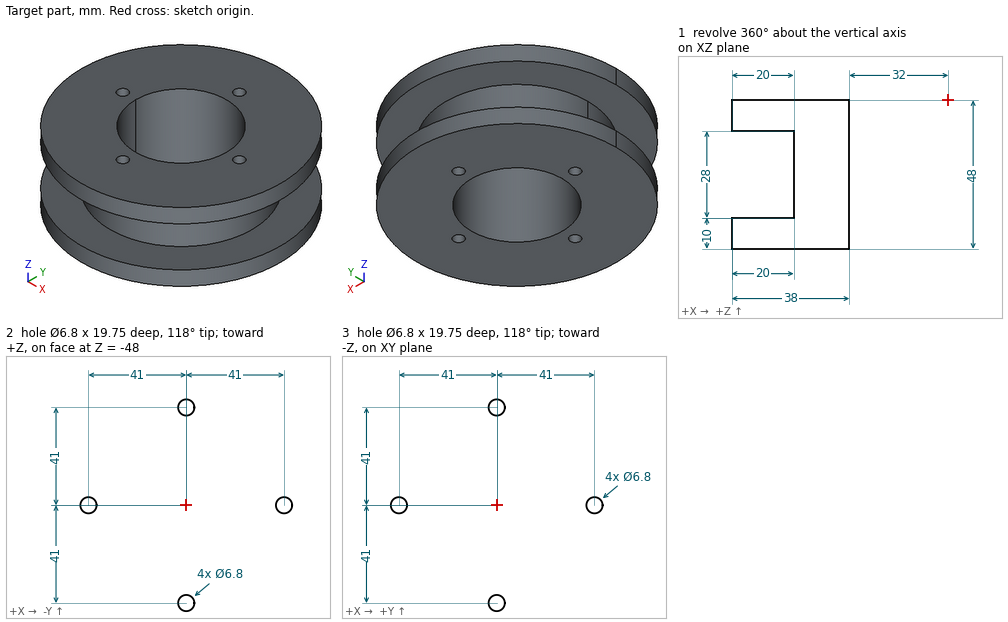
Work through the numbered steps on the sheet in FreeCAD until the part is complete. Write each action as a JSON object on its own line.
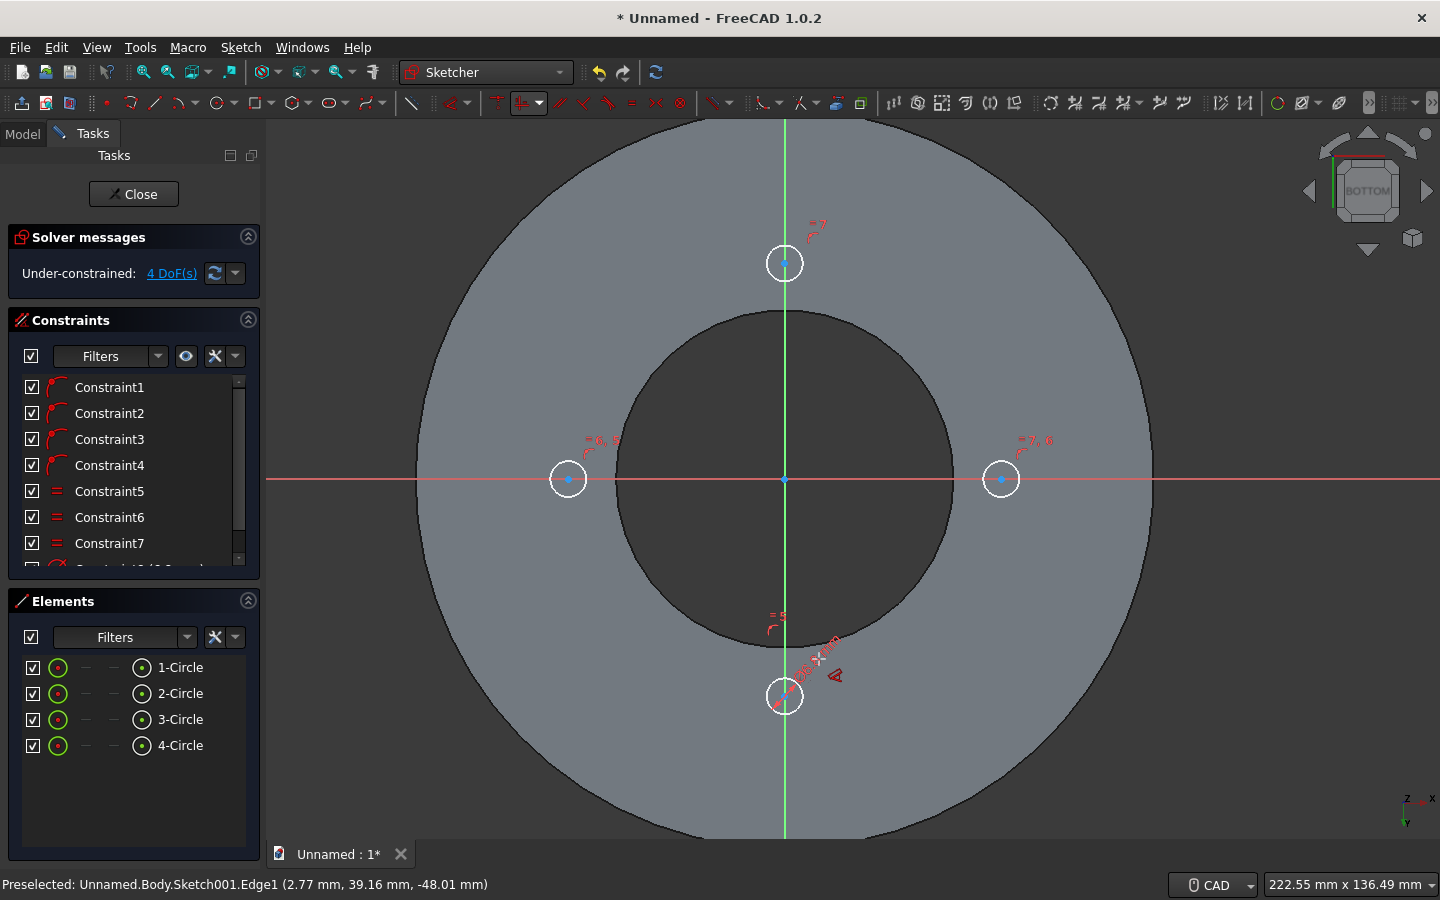
{"action": "left_click", "coordinate": [785, 696]}
{"action": "left_click", "coordinate": [819, 588]}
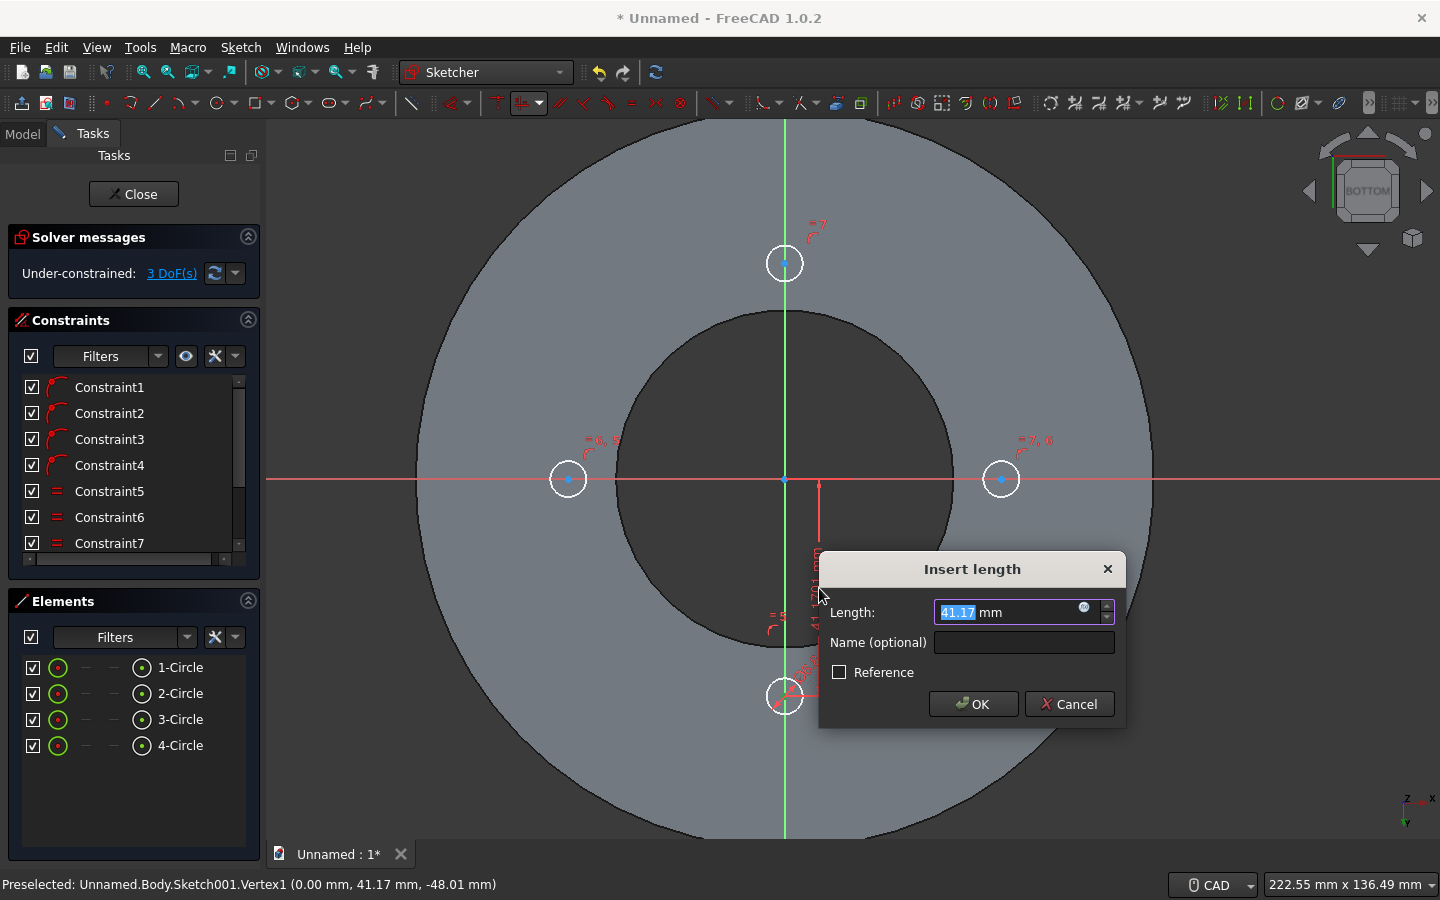
{"action": "type", "text": "41"}
{"action": "key", "text": "Return"}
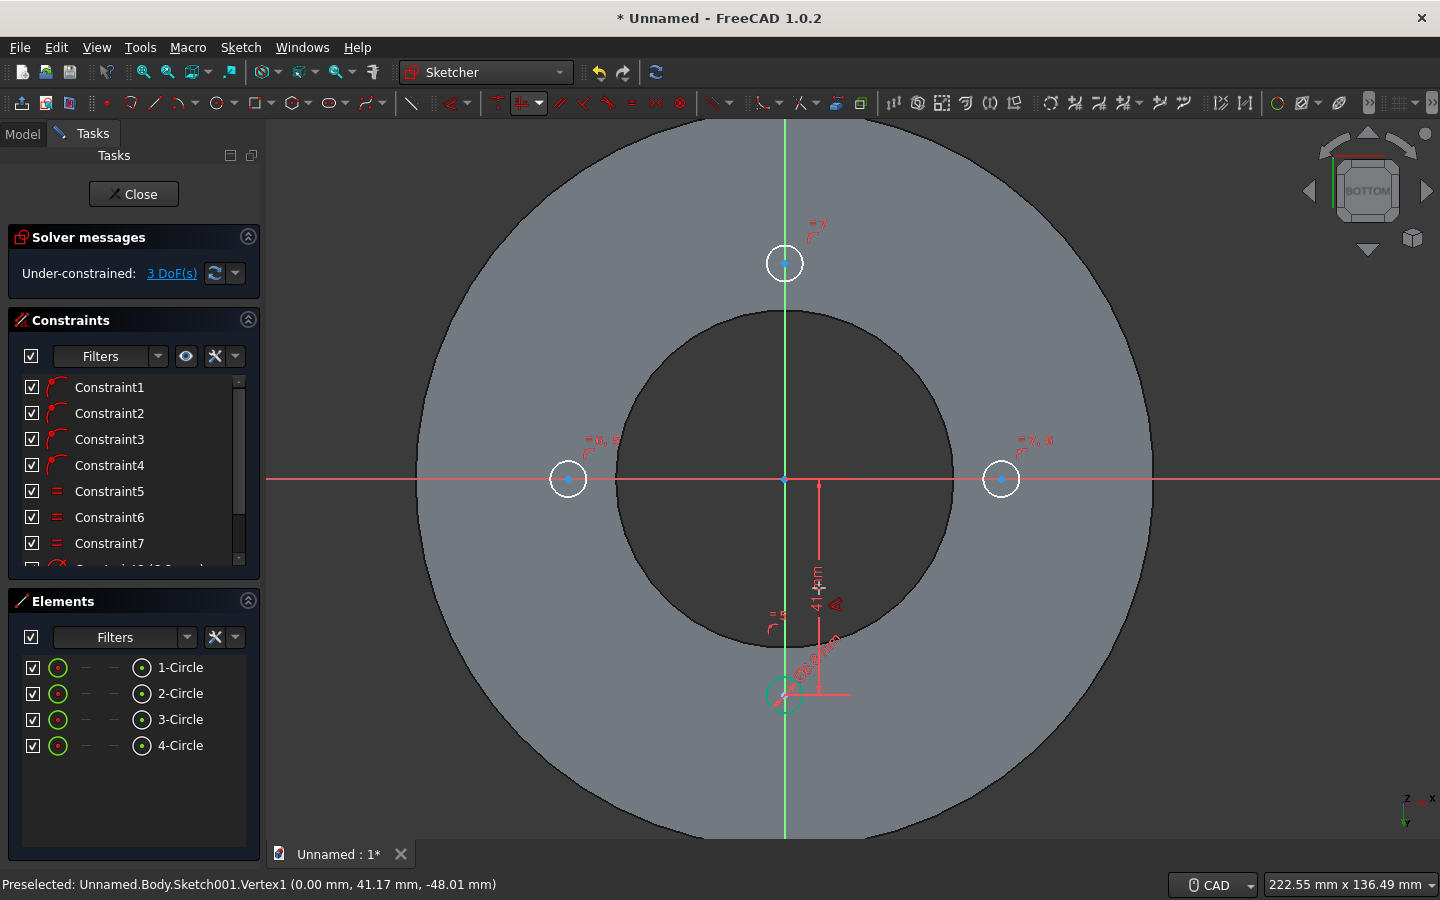
{"action": "left_click", "coordinate": [568, 479]}
{"action": "left_click", "coordinate": [677, 513]}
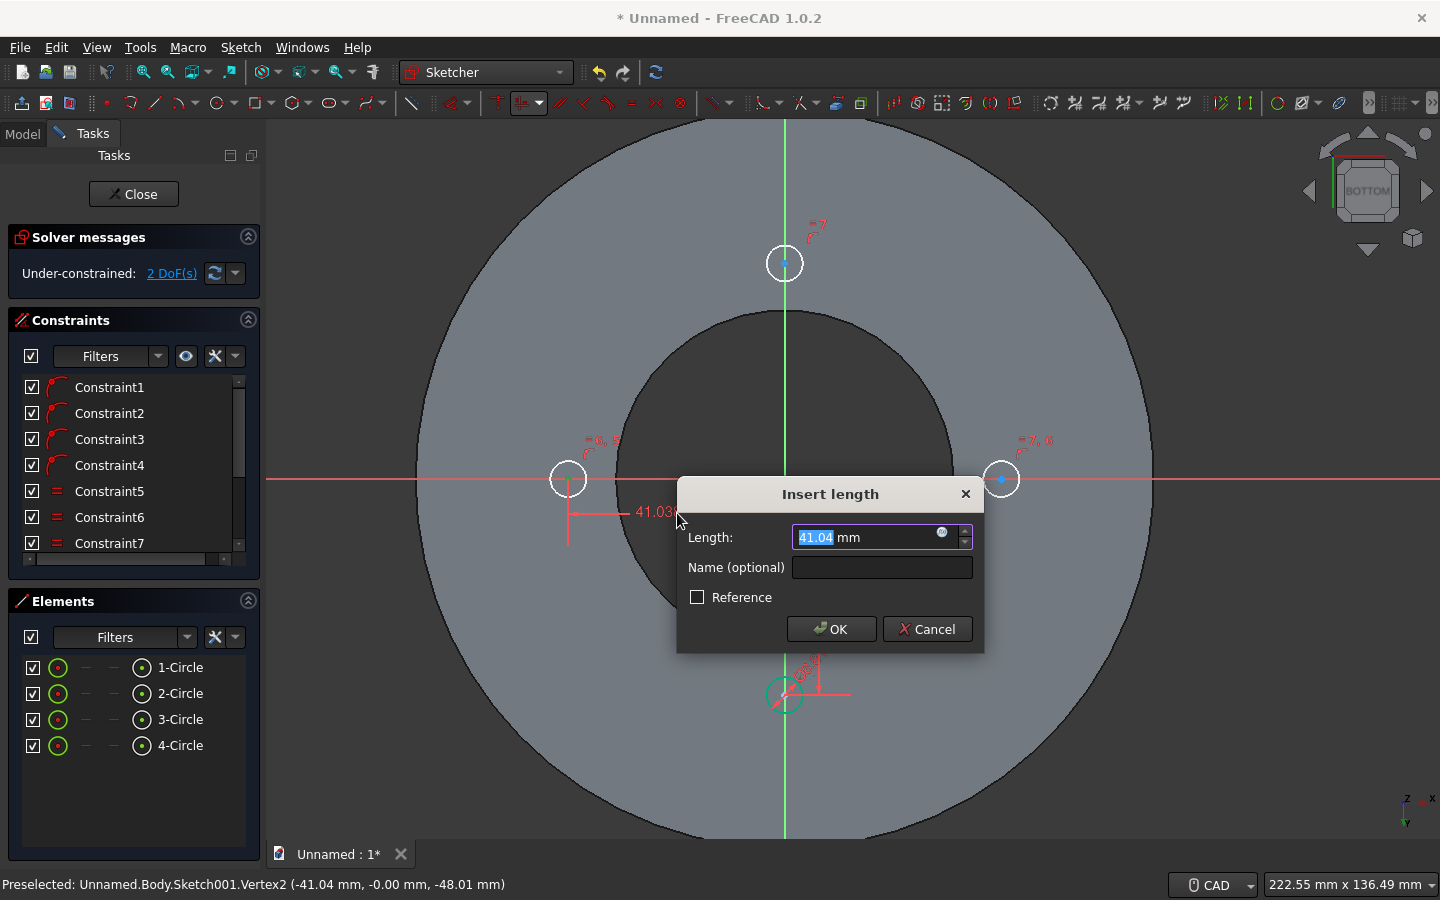
{"action": "type", "text": "41"}
{"action": "key", "text": "Return"}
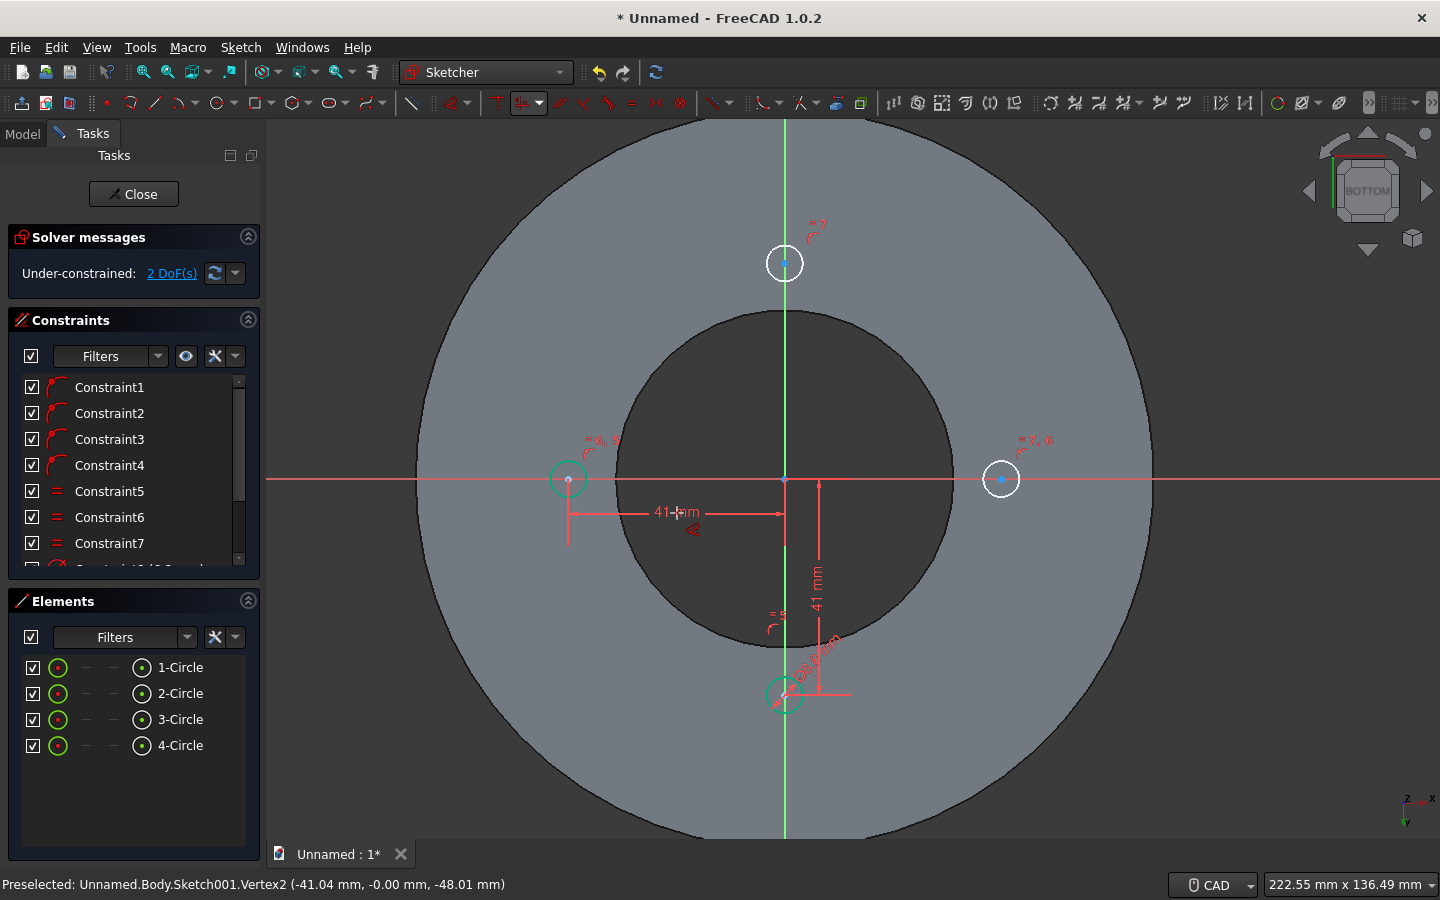
{"action": "left_click", "coordinate": [1001, 479]}
{"action": "left_click", "coordinate": [893, 513]}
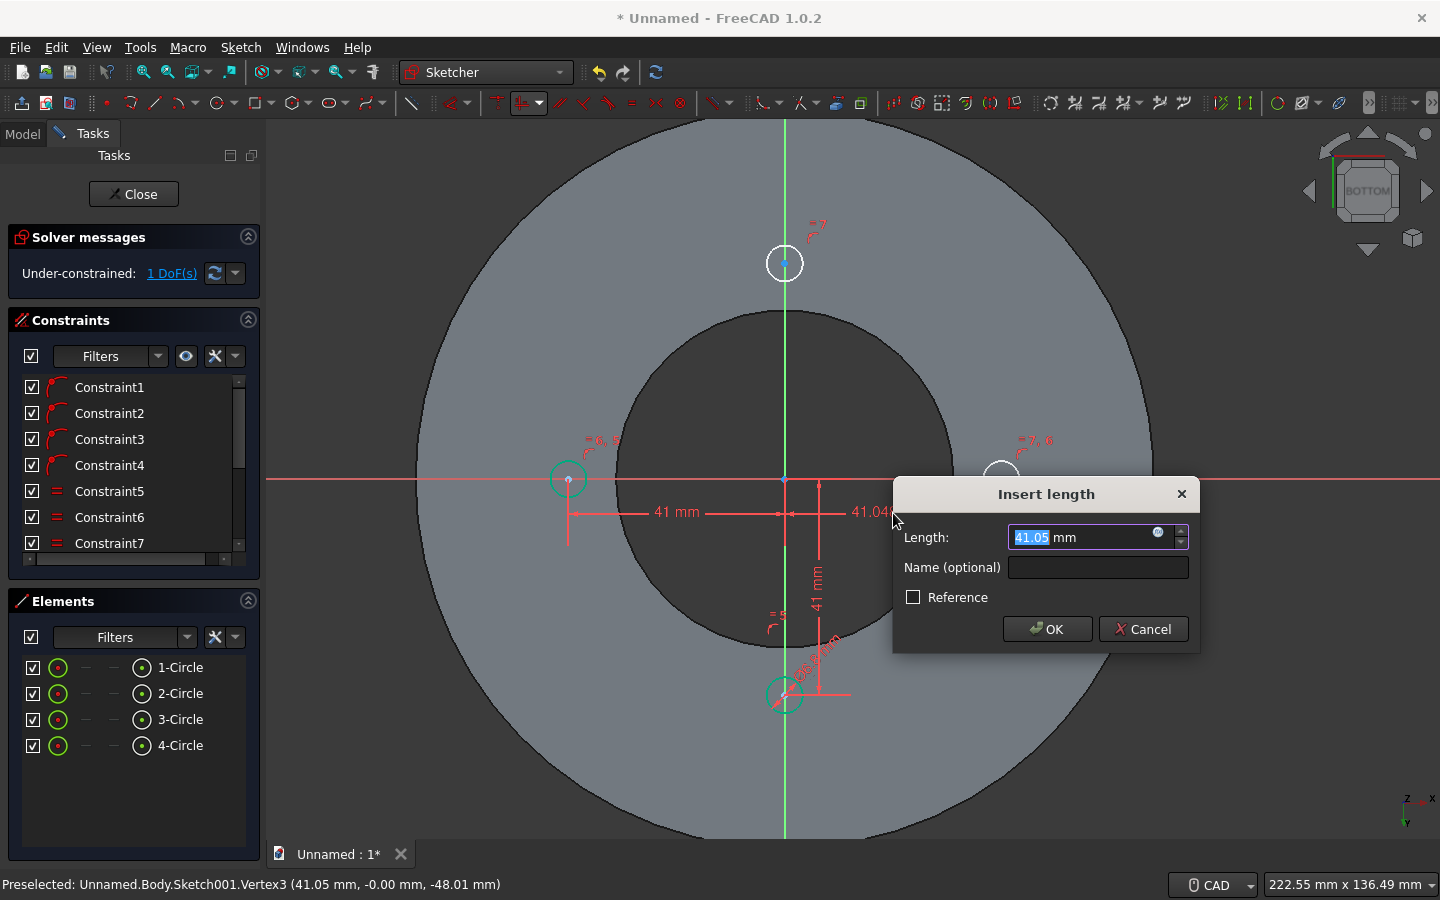
{"action": "type", "text": "41"}
{"action": "key", "text": "Return"}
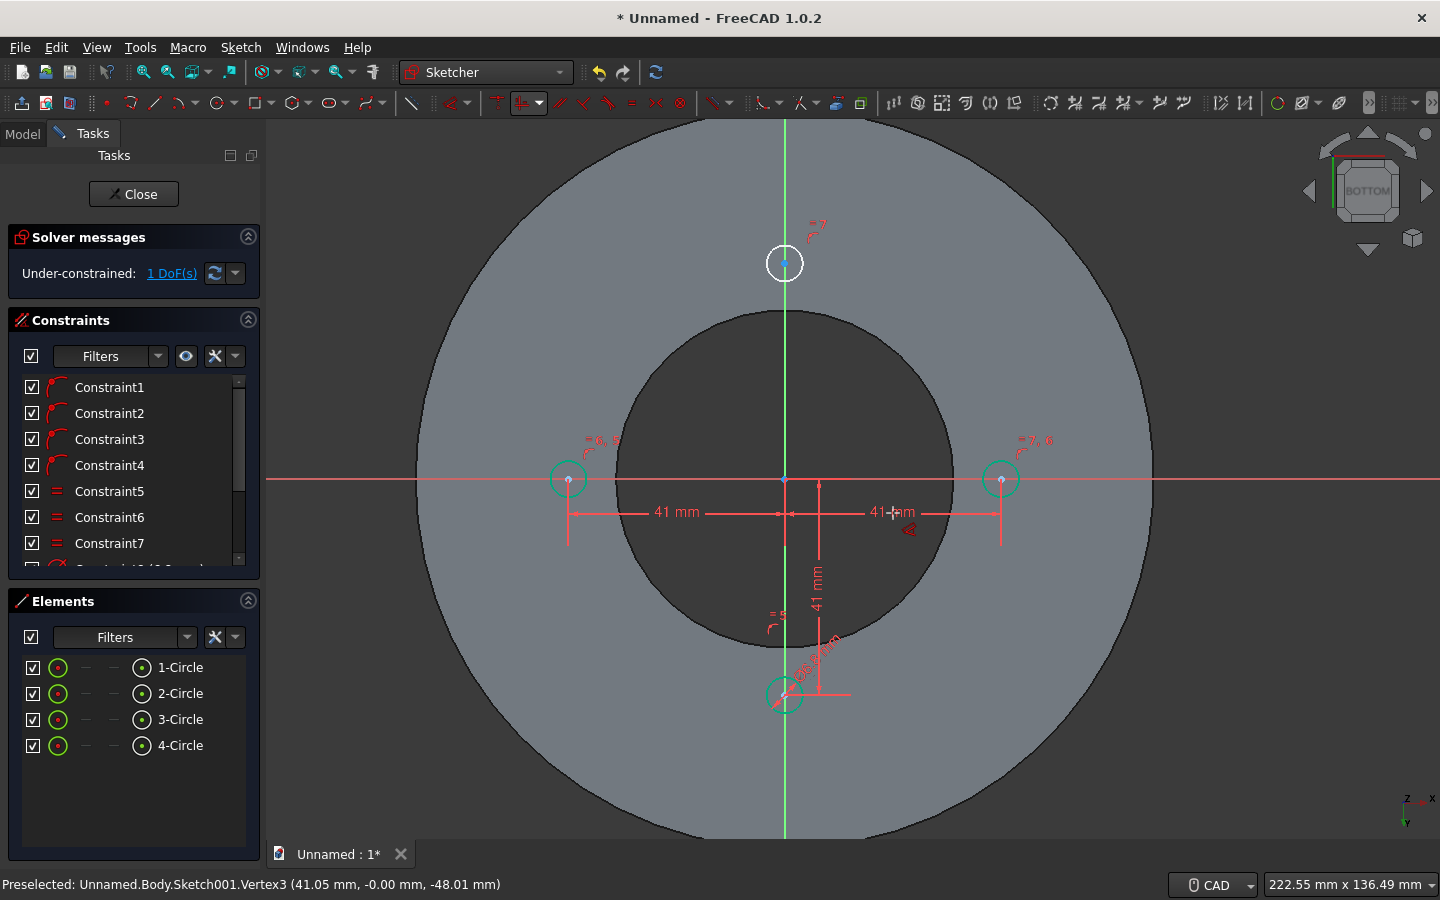
{"action": "left_click", "coordinate": [785, 263]}
{"action": "left_click", "coordinate": [819, 371]}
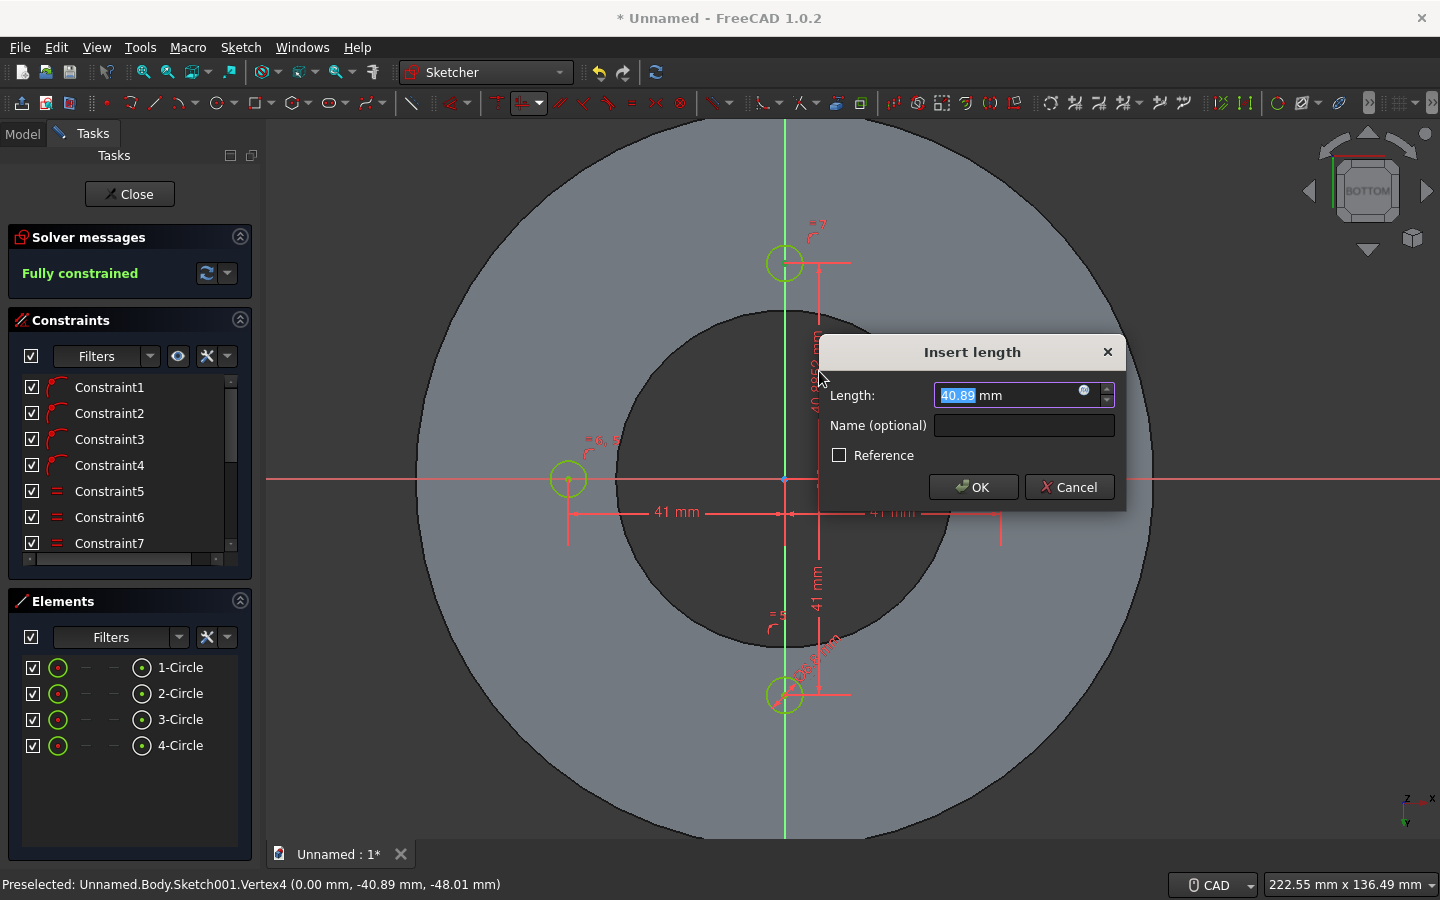
{"action": "type", "text": "41"}
{"action": "key", "text": "Return"}
{"action": "key", "text": "Escape"}